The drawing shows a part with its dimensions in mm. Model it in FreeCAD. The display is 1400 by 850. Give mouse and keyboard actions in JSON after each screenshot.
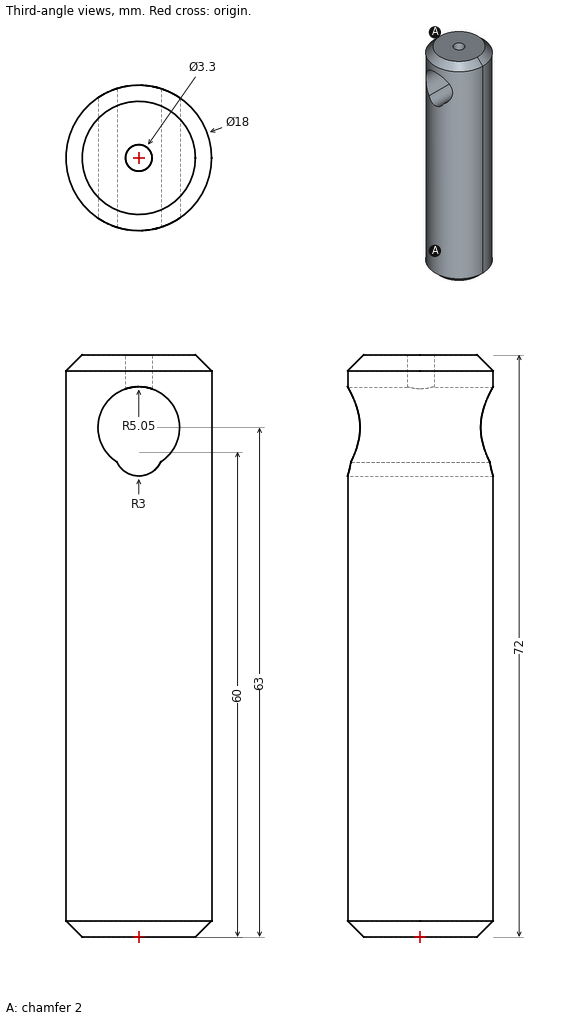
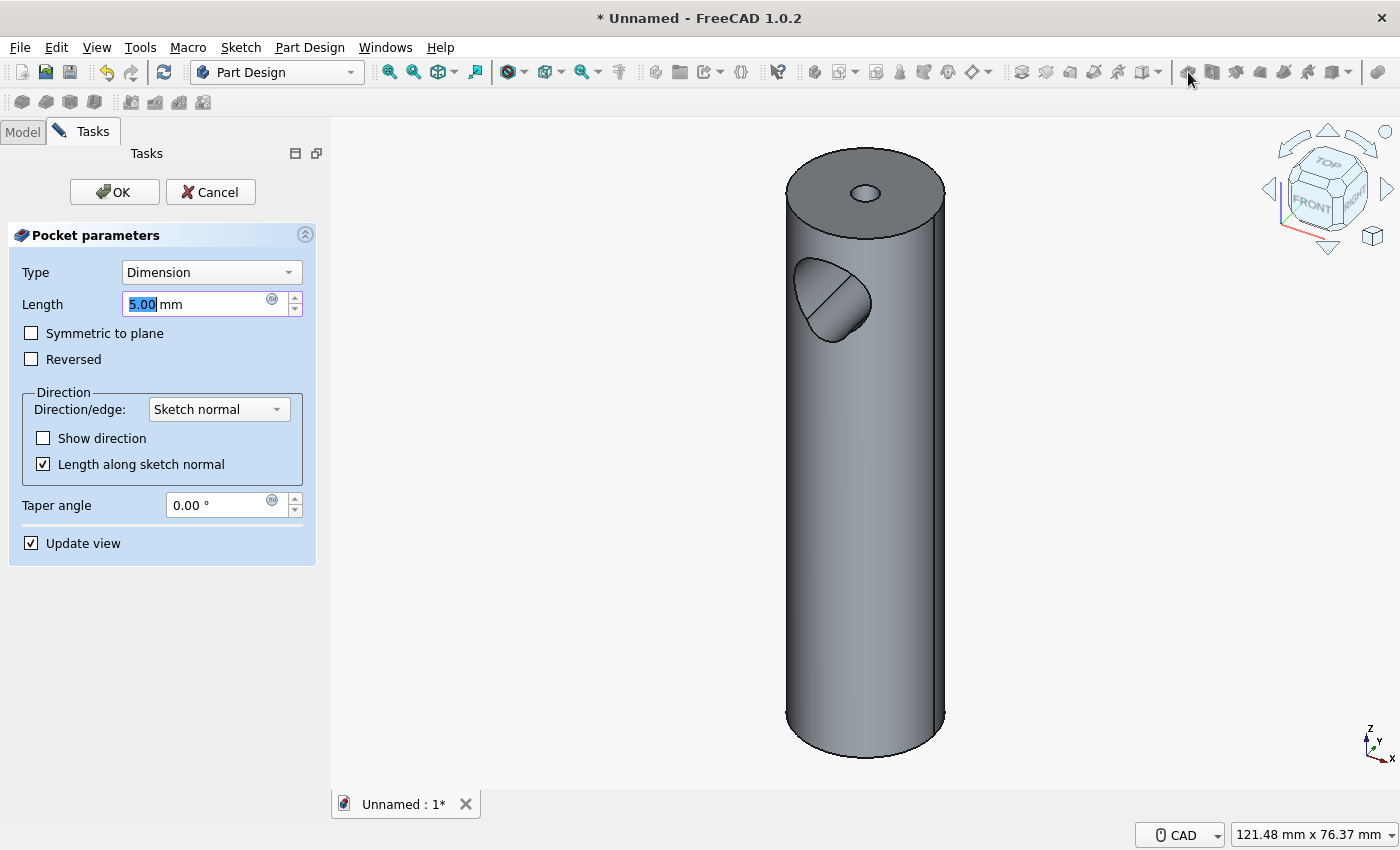
{"action": "left_click", "coordinate": [212, 272]}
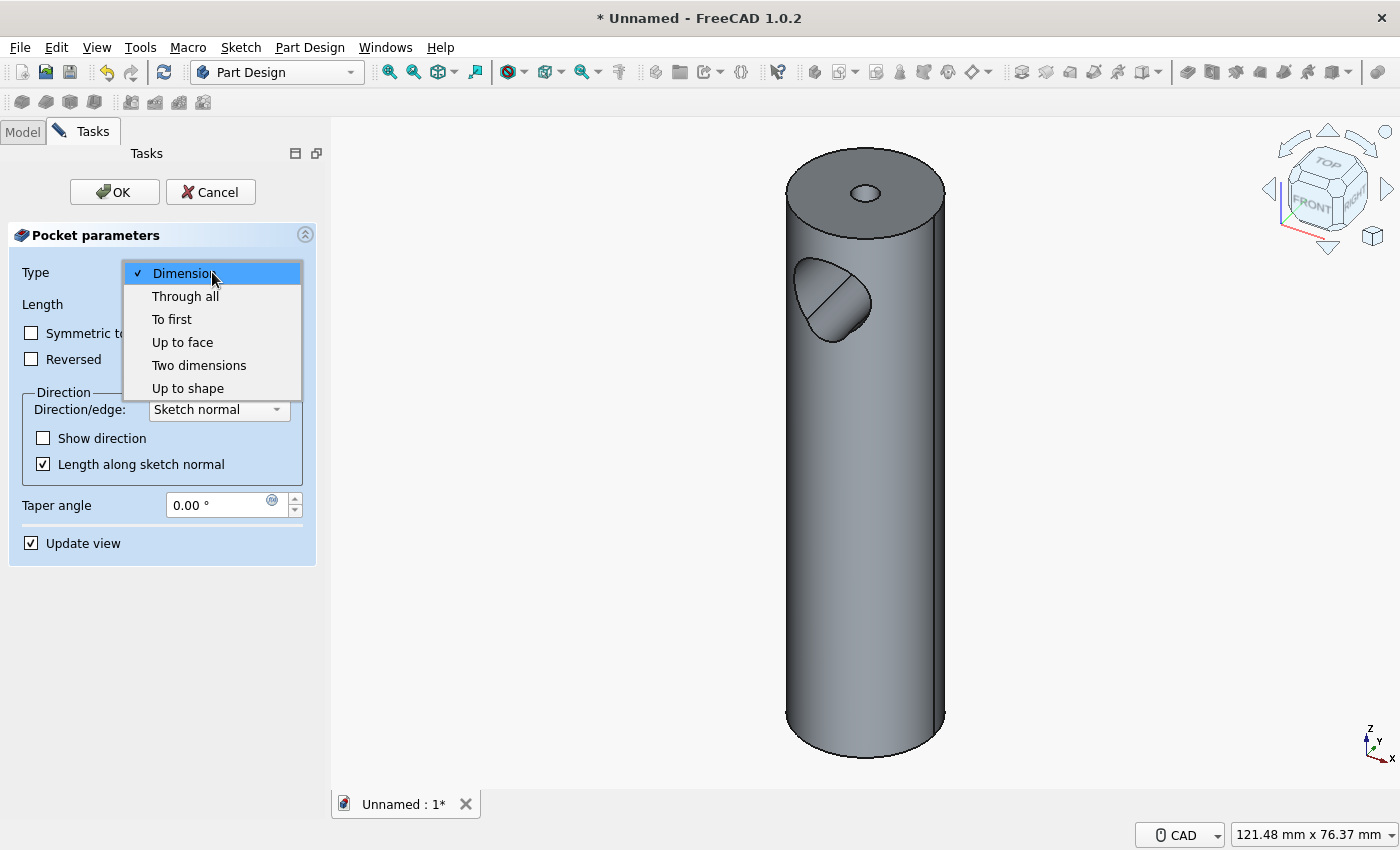
{"action": "left_click", "coordinate": [212, 320]}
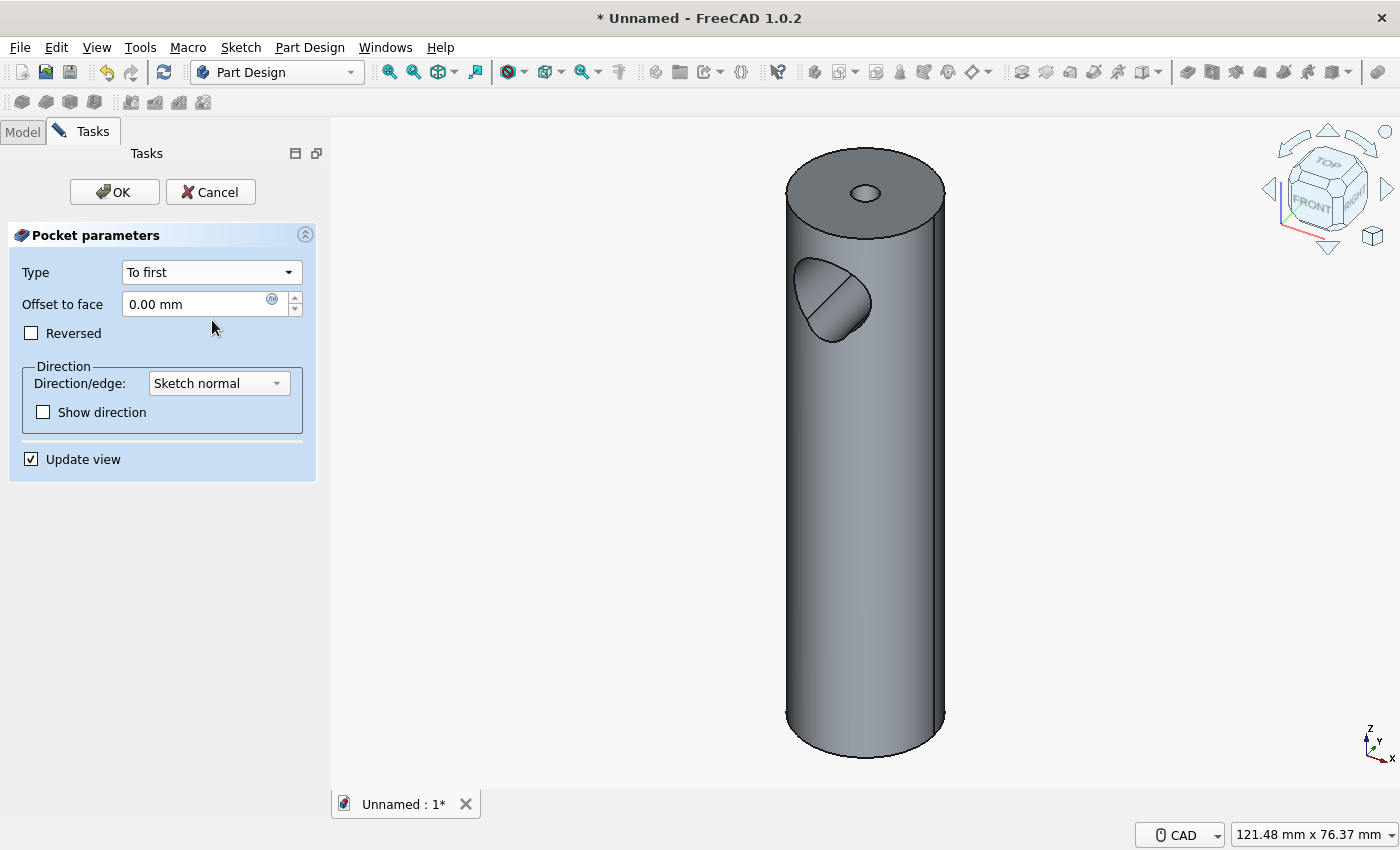
{"action": "left_click", "coordinate": [115, 192]}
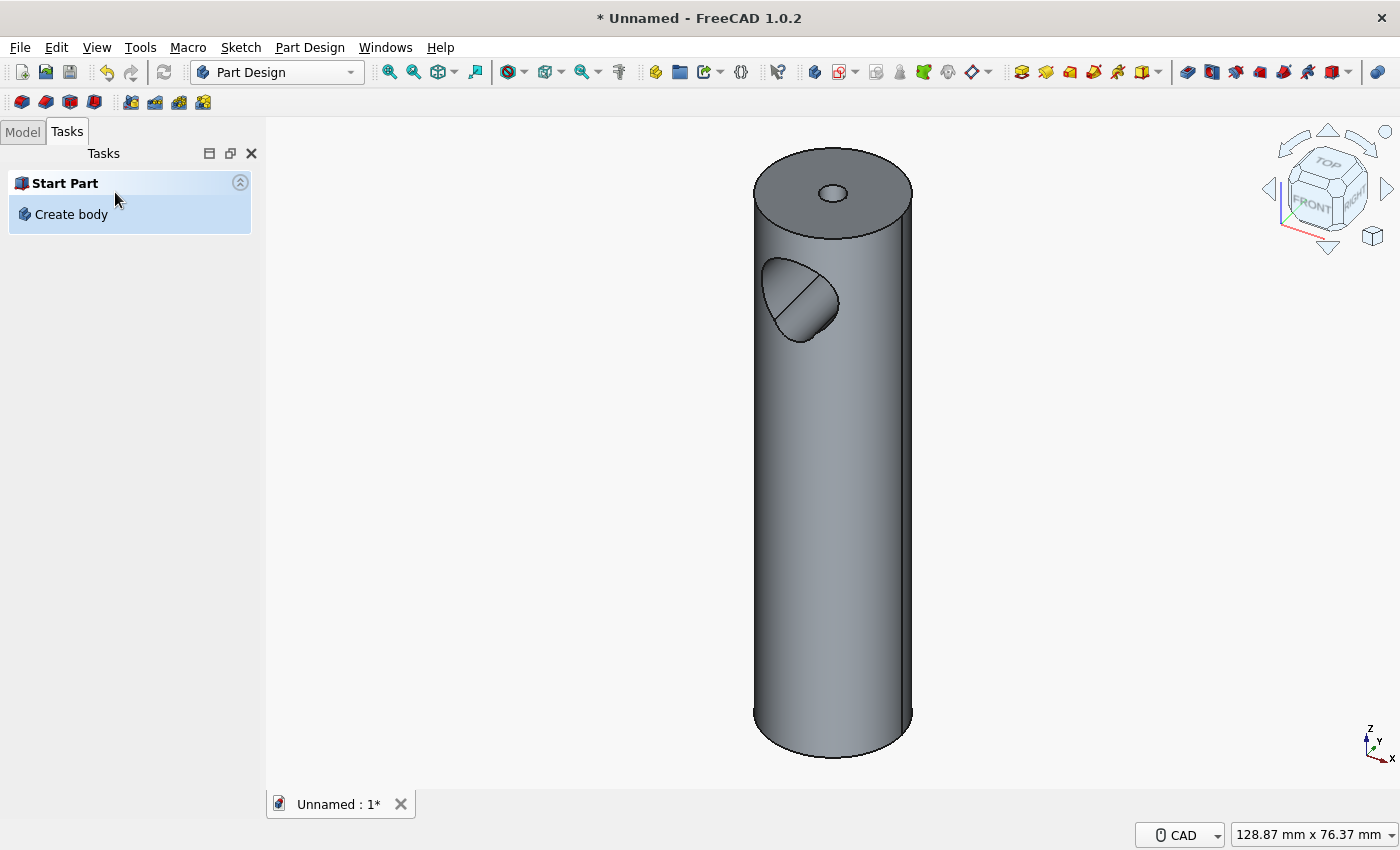
{"action": "left_click", "coordinate": [754, 197]}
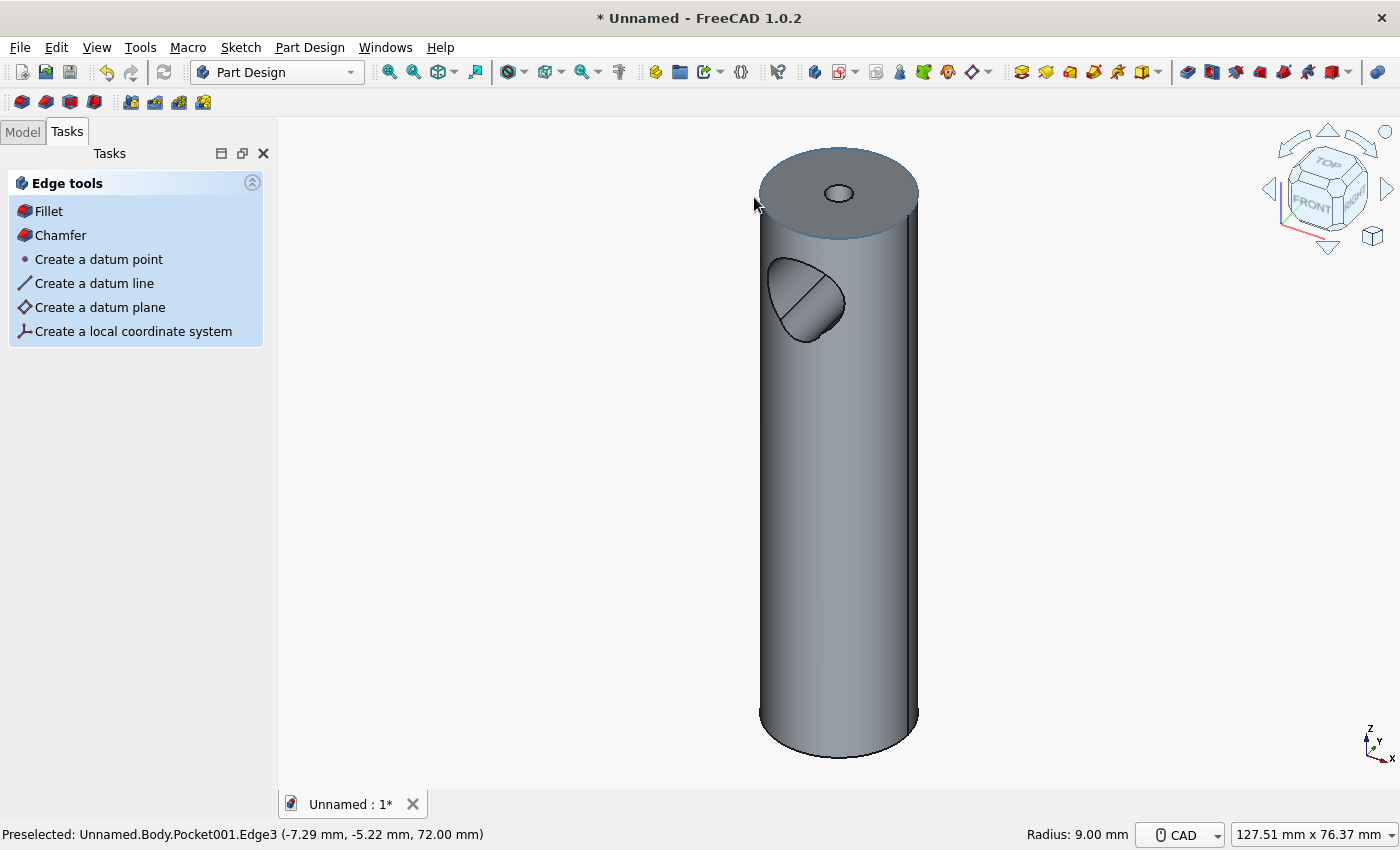
{"action": "key", "text": "0"}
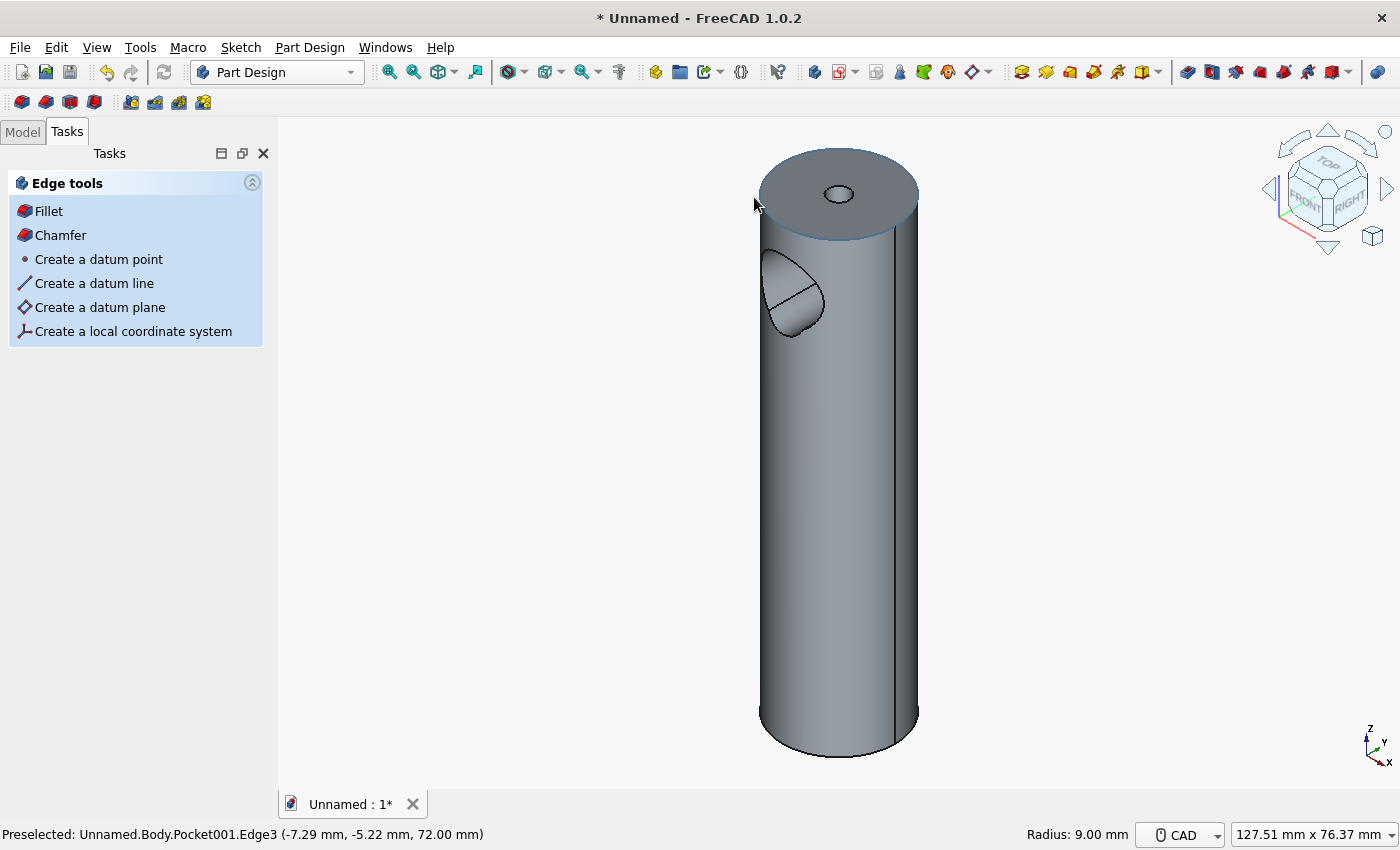
{"action": "key", "text": "2"}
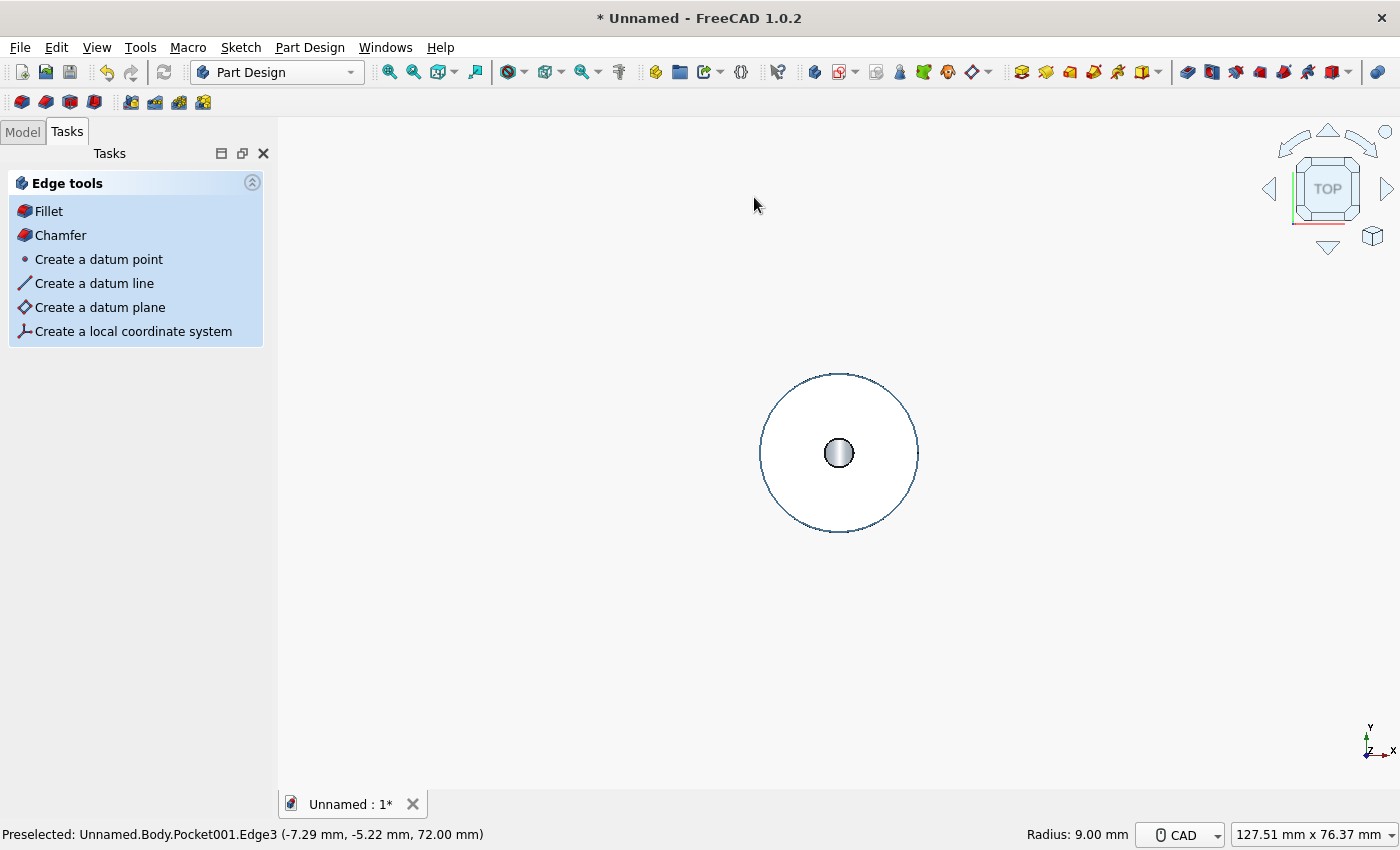
{"action": "left_click", "coordinate": [390, 72]}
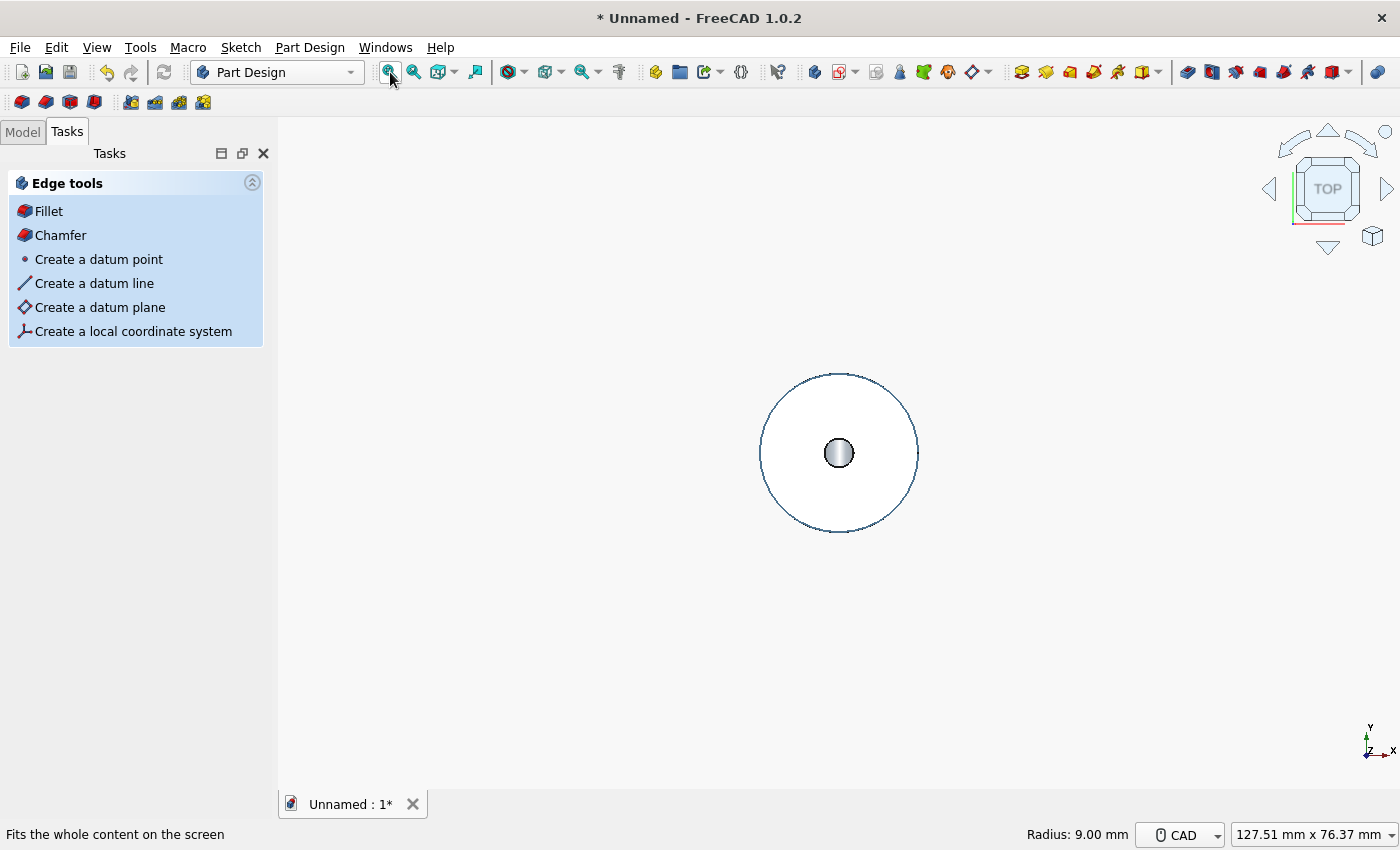
{"action": "key", "text": "1"}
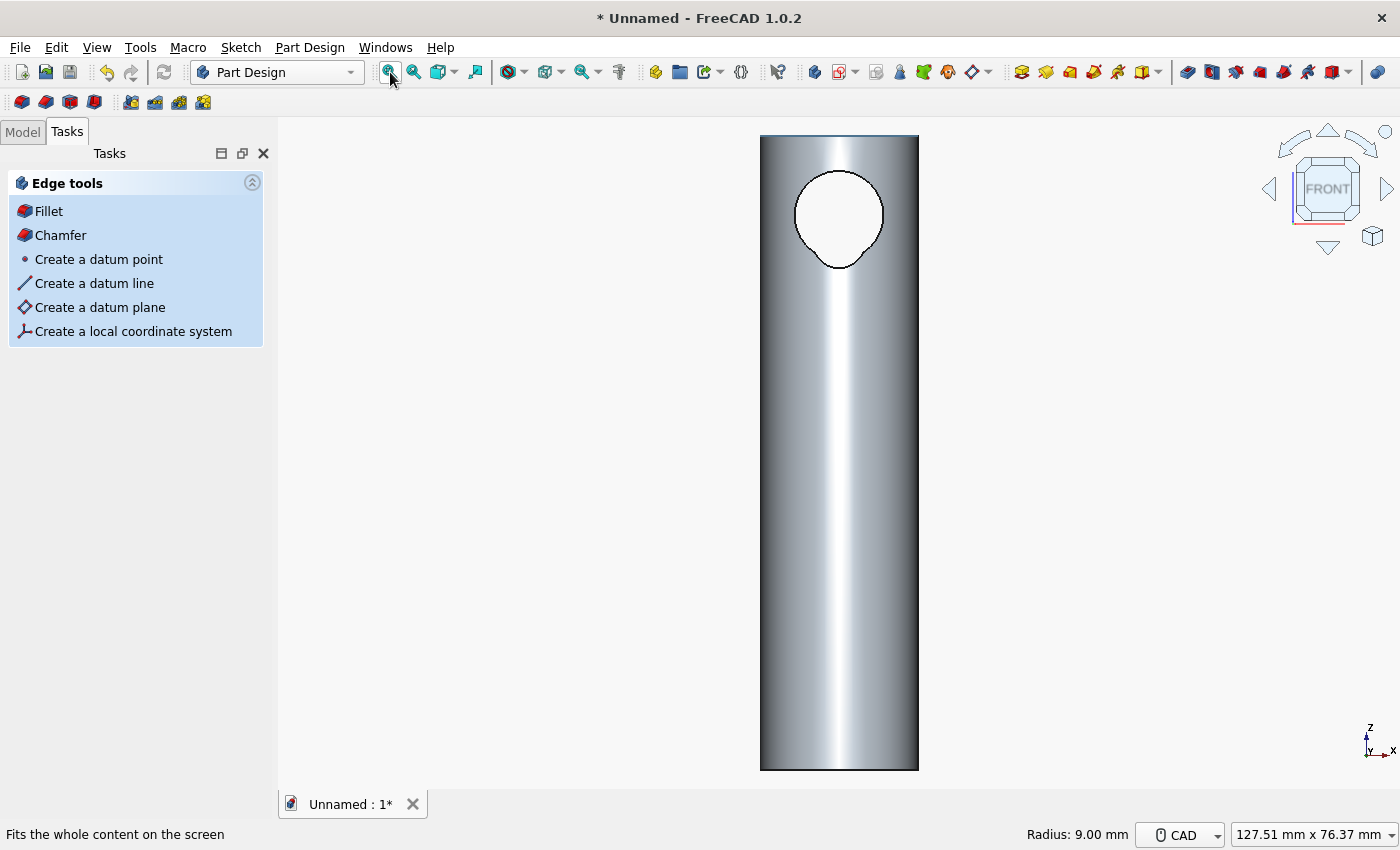
{"action": "key", "text": "3"}